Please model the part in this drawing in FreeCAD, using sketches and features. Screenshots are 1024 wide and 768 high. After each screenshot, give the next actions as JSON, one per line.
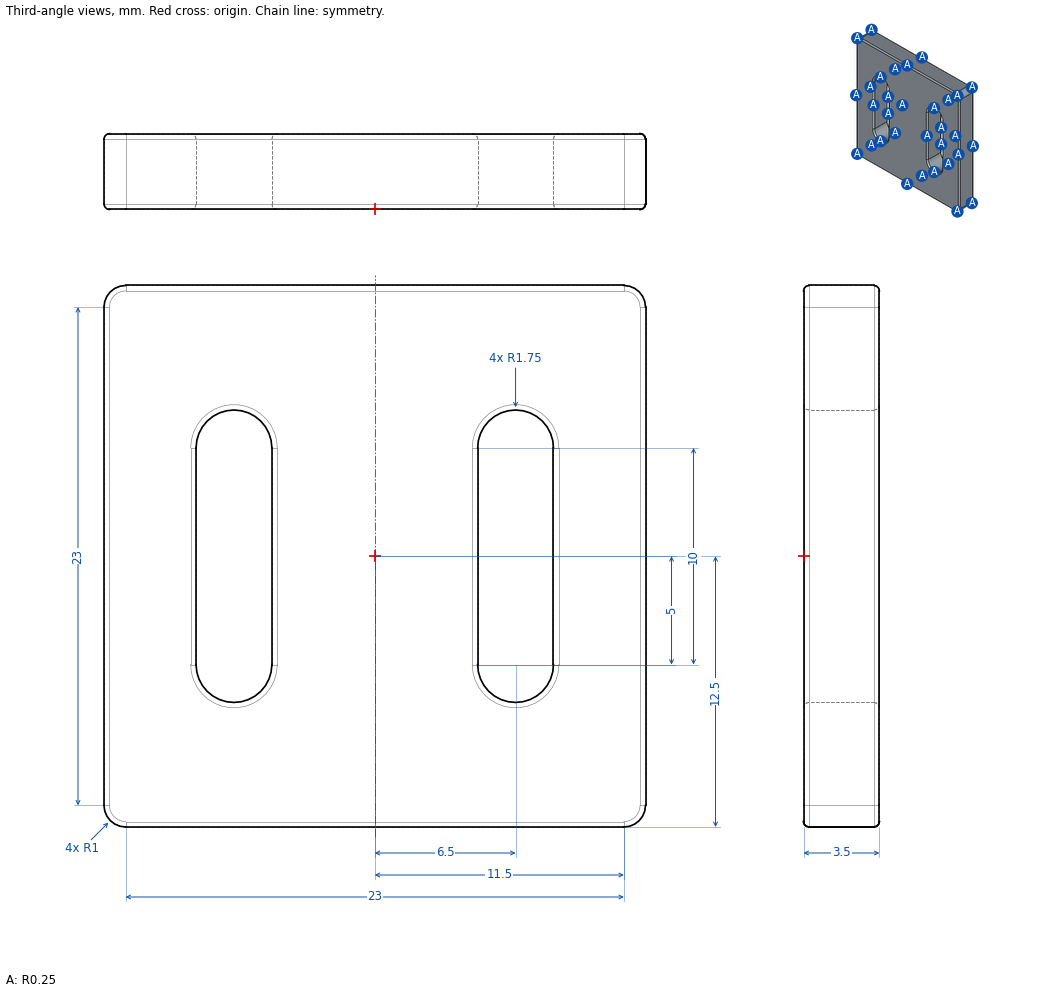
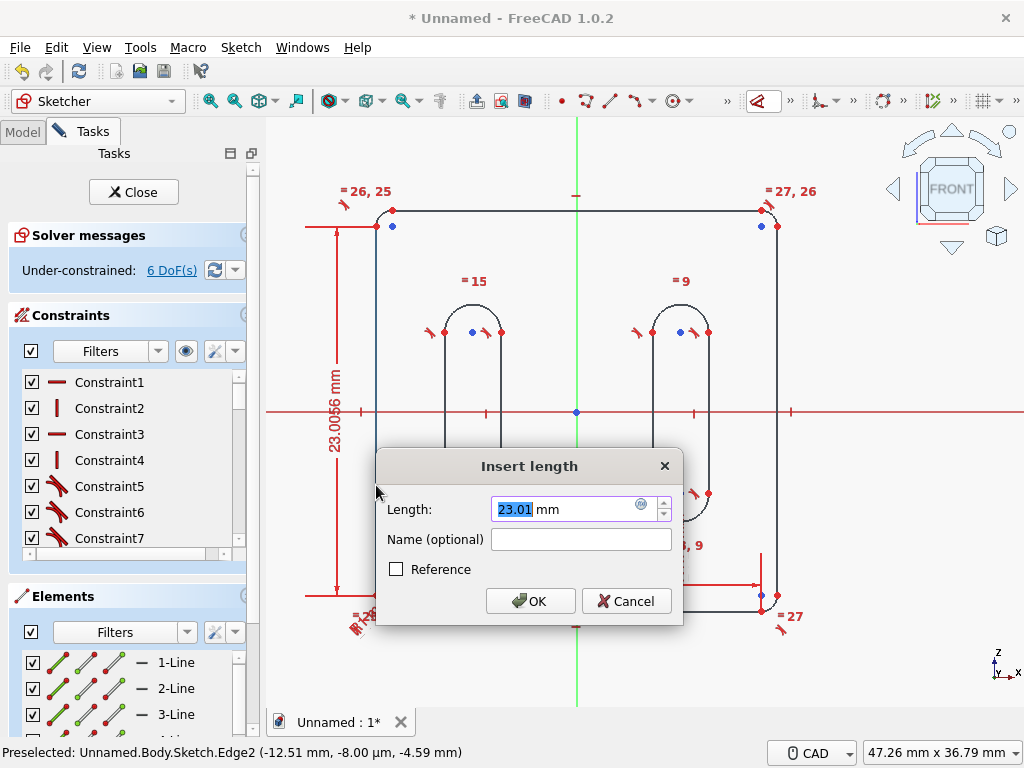
{"action": "type", "text": "23"}
{"action": "key", "text": "Return"}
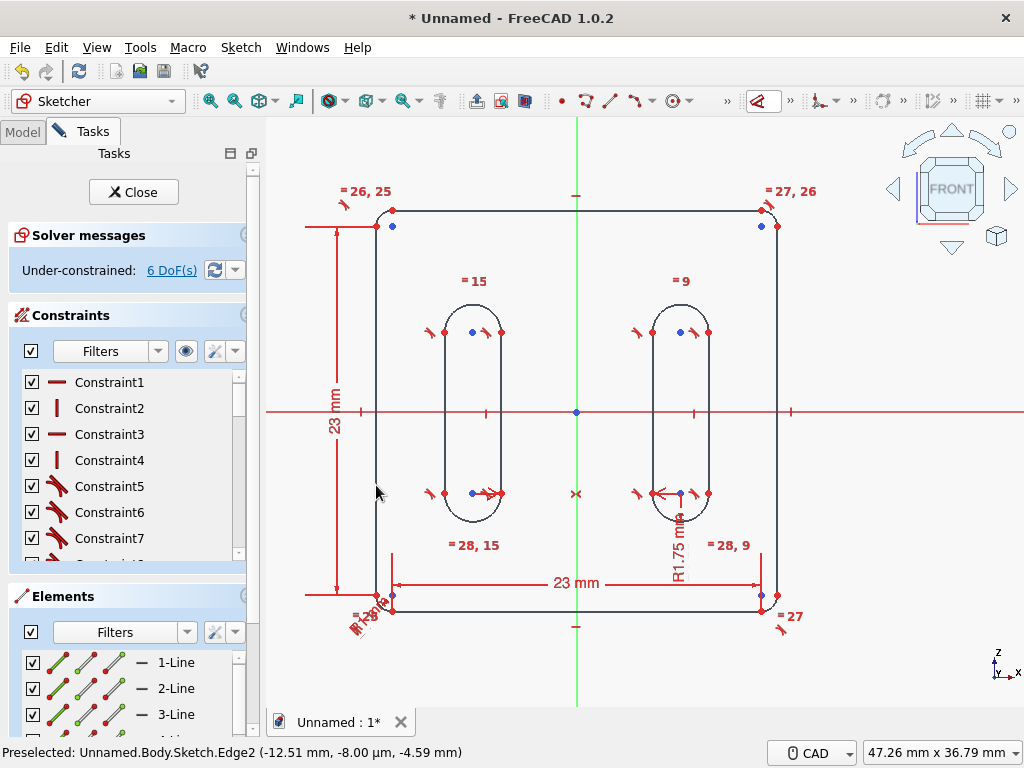
{"action": "left_click", "coordinate": [653, 445]}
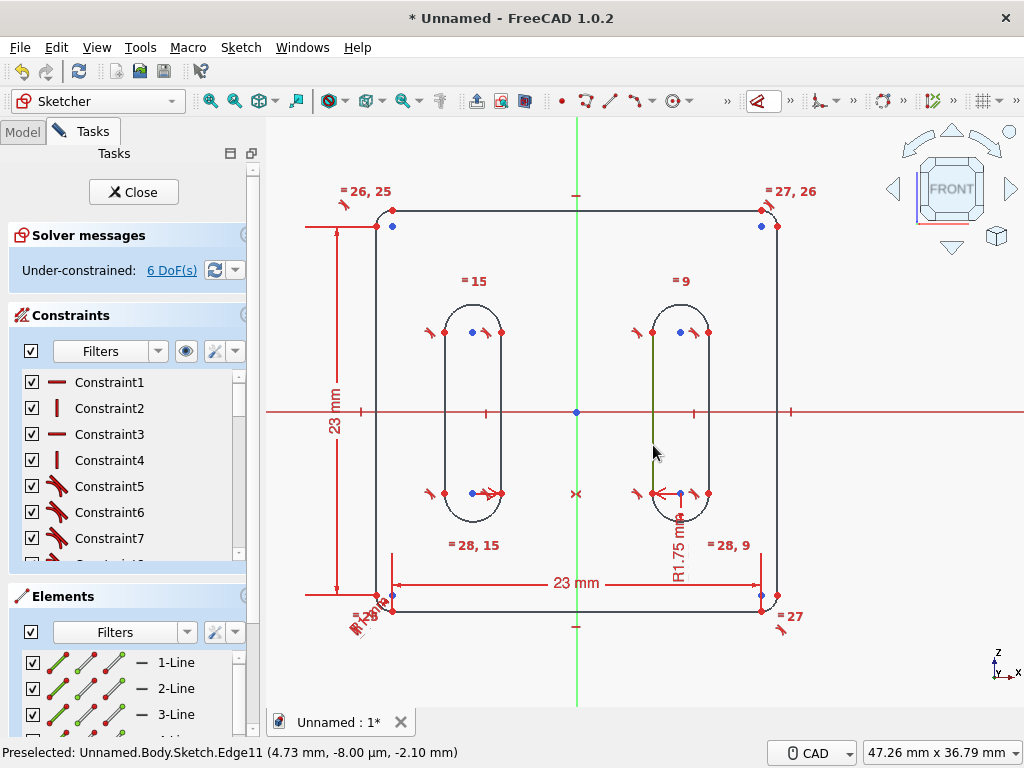
{"action": "key", "text": "i"}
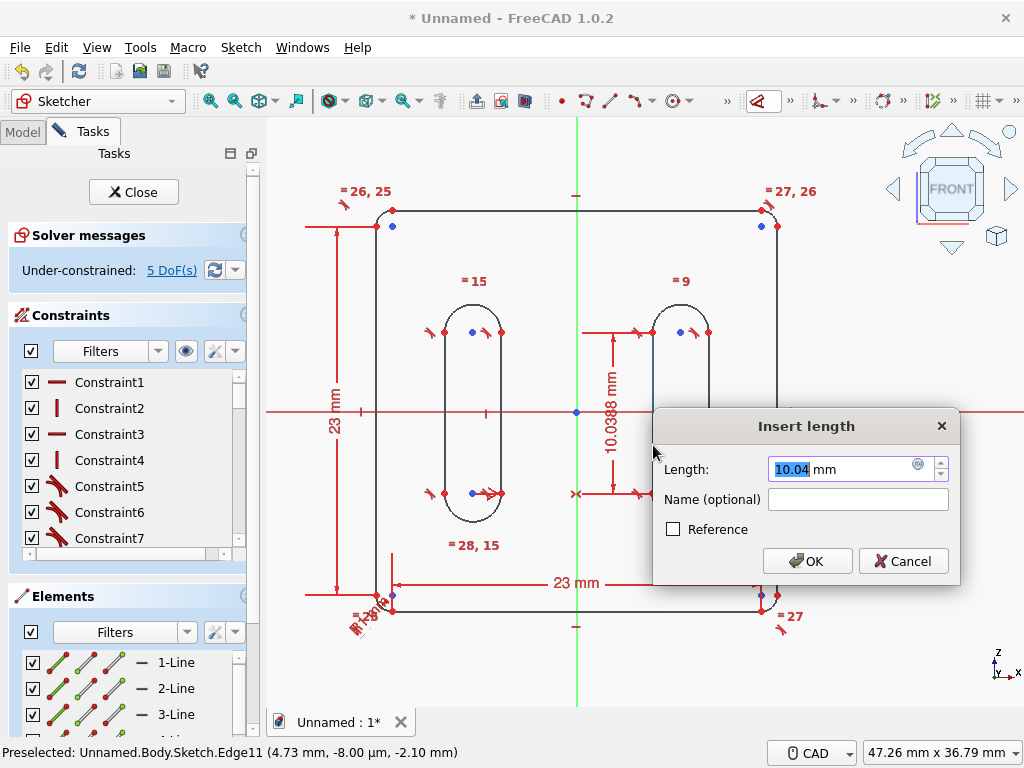
{"action": "type", "text": "10"}
{"action": "key", "text": "Return"}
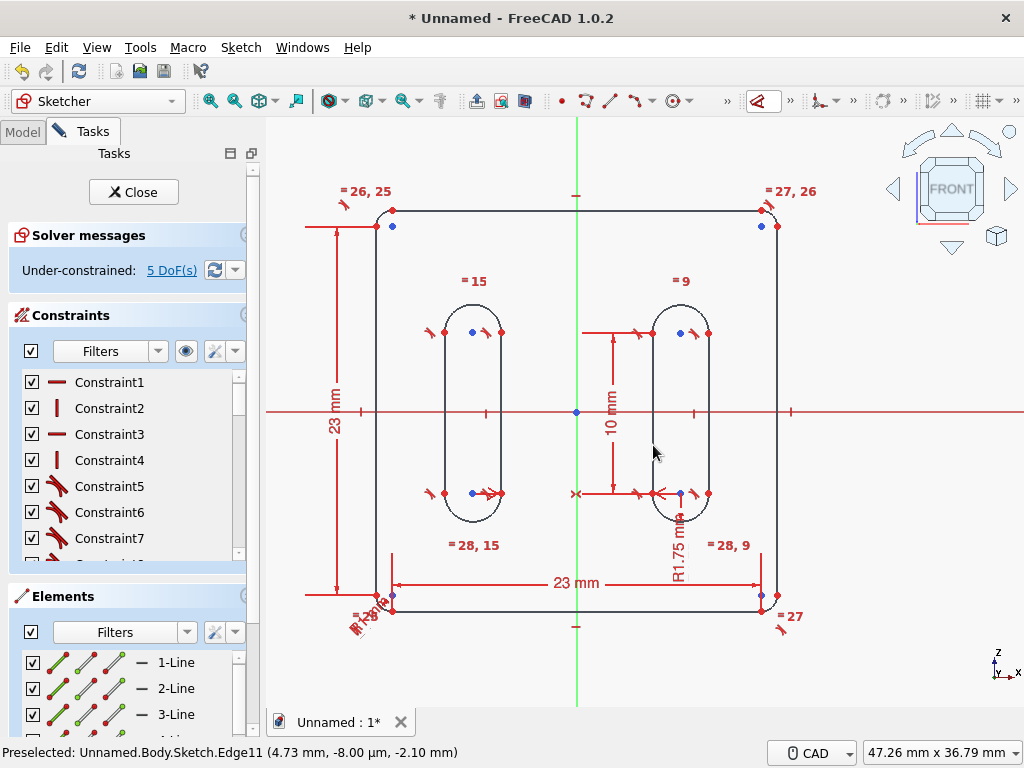
{"action": "left_click", "coordinate": [445, 445]}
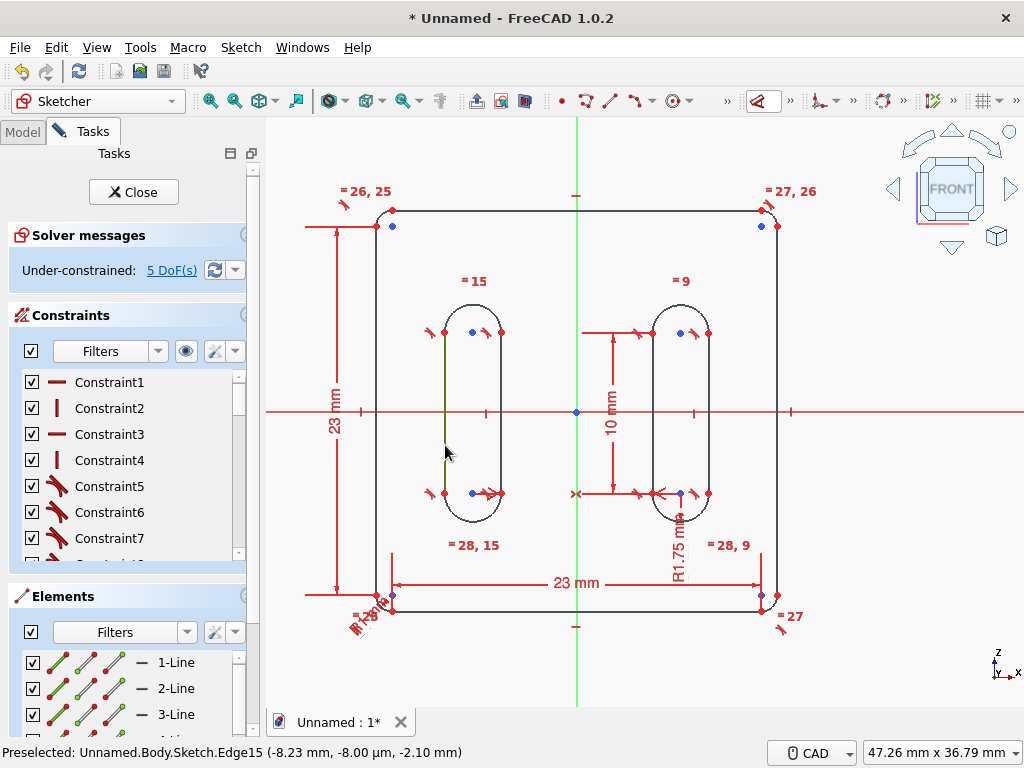
{"action": "key", "text": "i"}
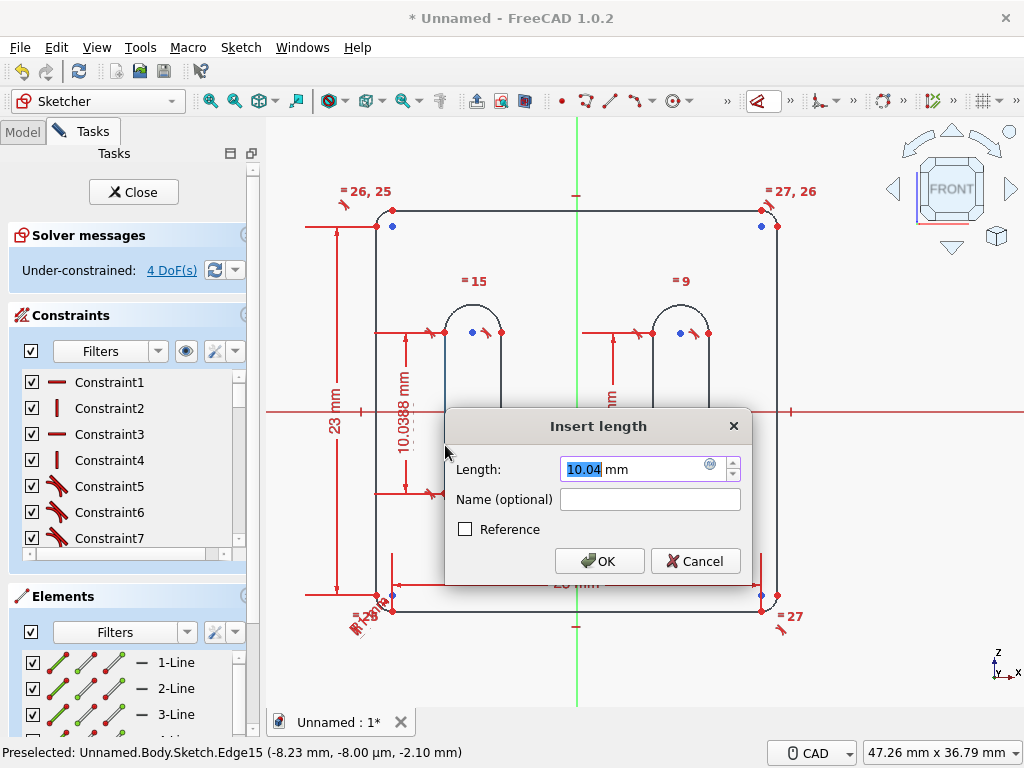
{"action": "type", "text": "10"}
{"action": "key", "text": "Return"}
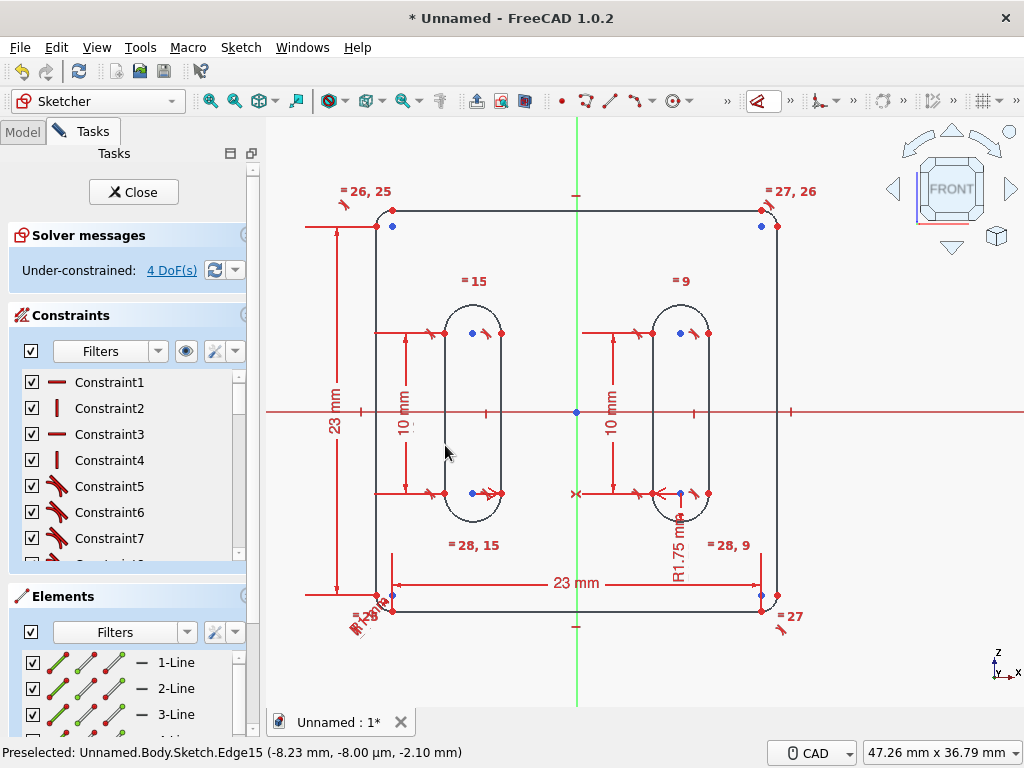
{"action": "left_click", "coordinate": [653, 494]}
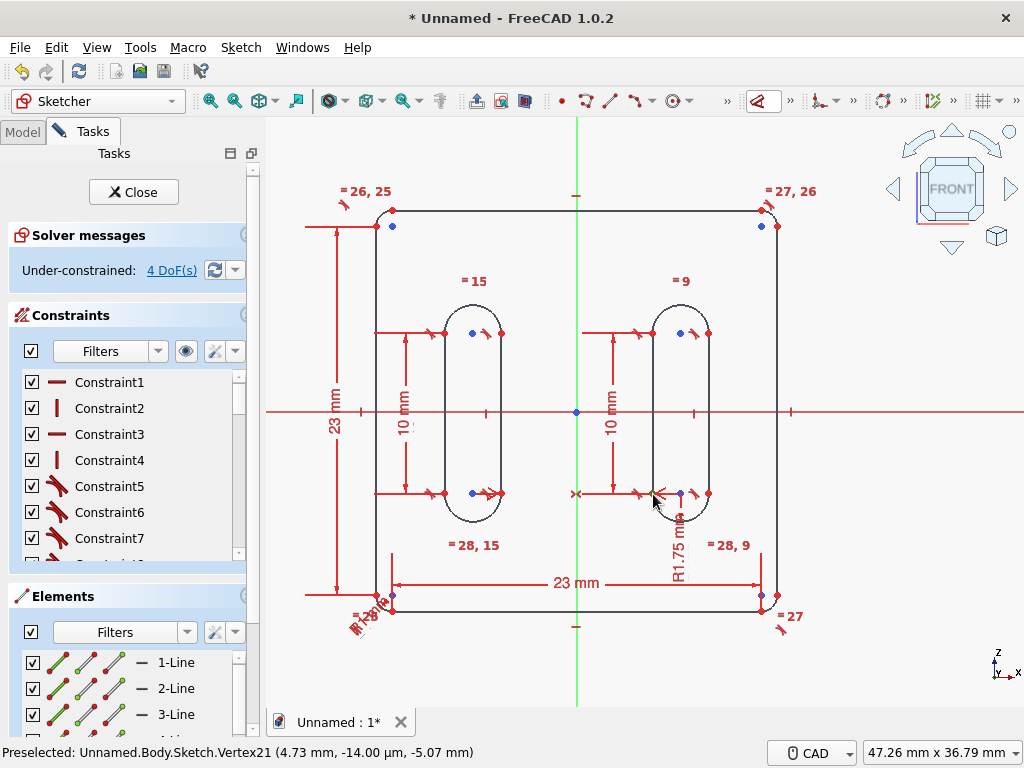
{"action": "left_click", "coordinate": [776, 102]}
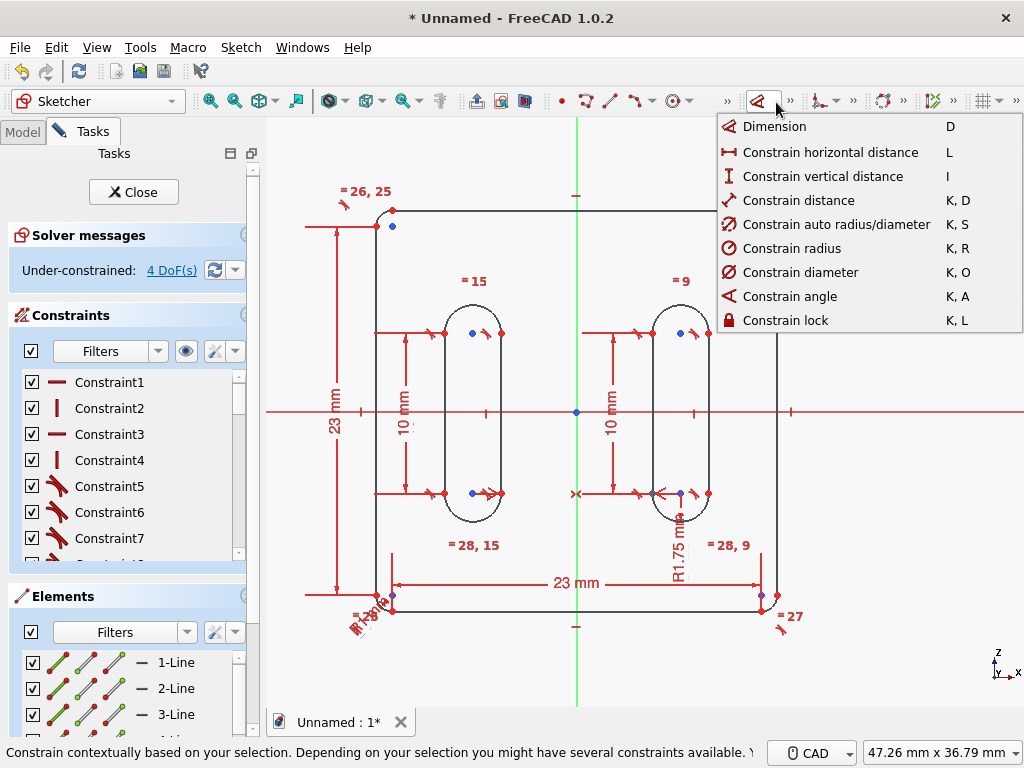
{"action": "left_click", "coordinate": [870, 176]}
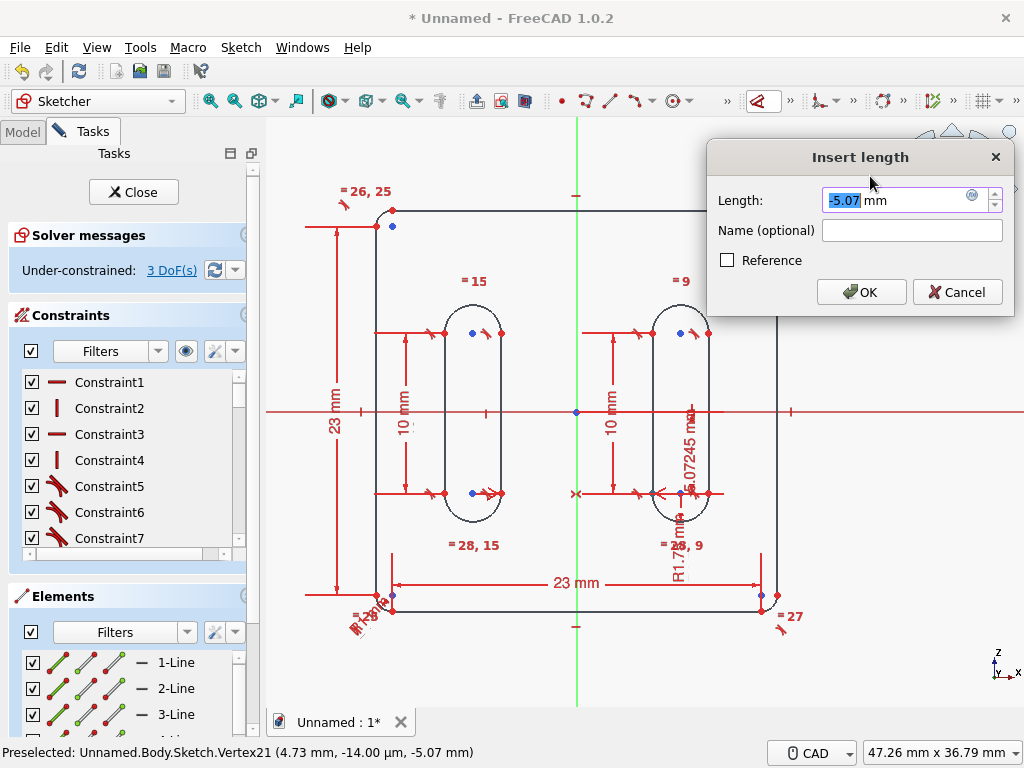
{"action": "type", "text": "-5"}
{"action": "key", "text": "Return"}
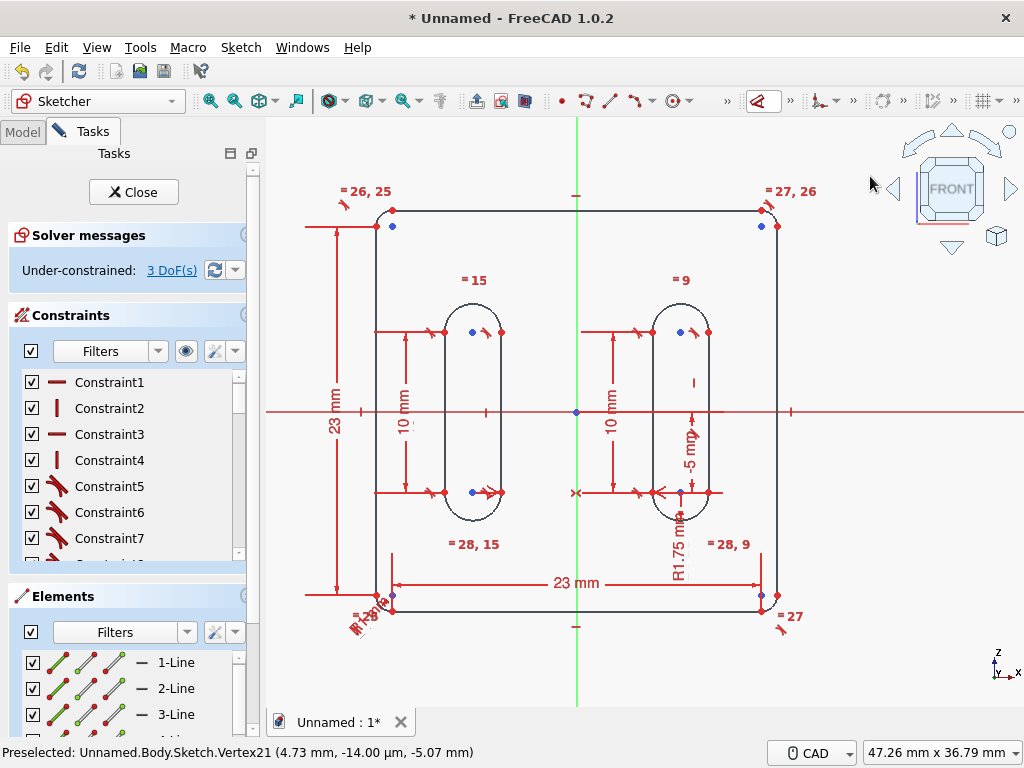
{"action": "left_click", "coordinate": [681, 493]}